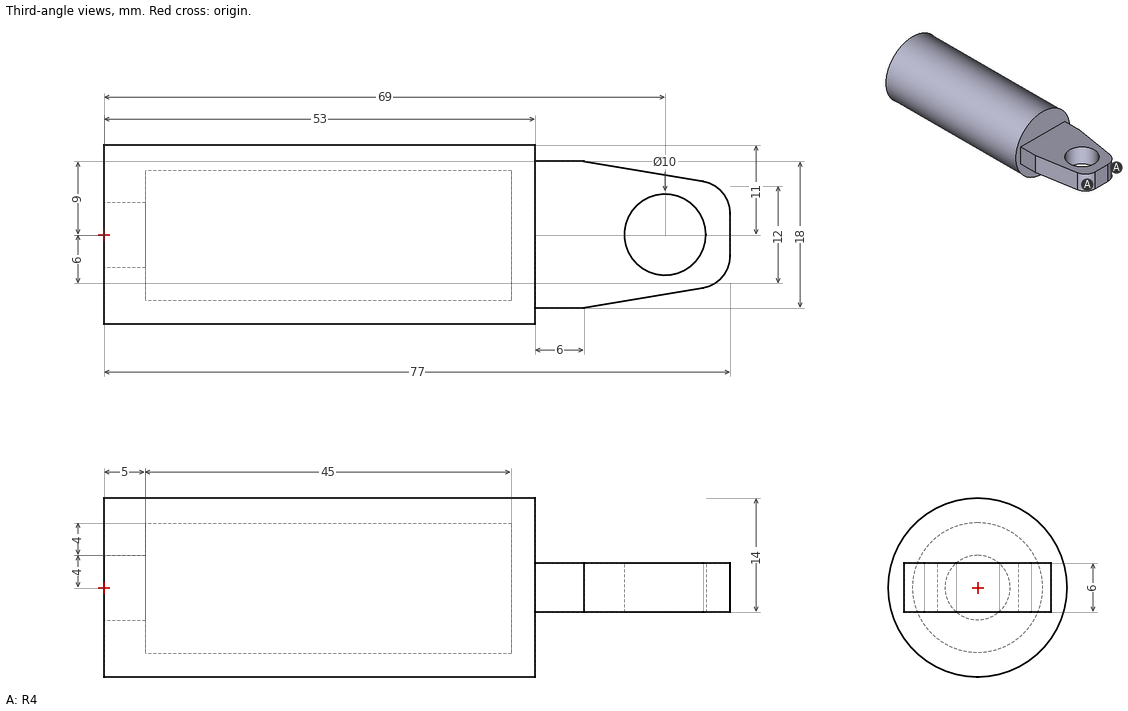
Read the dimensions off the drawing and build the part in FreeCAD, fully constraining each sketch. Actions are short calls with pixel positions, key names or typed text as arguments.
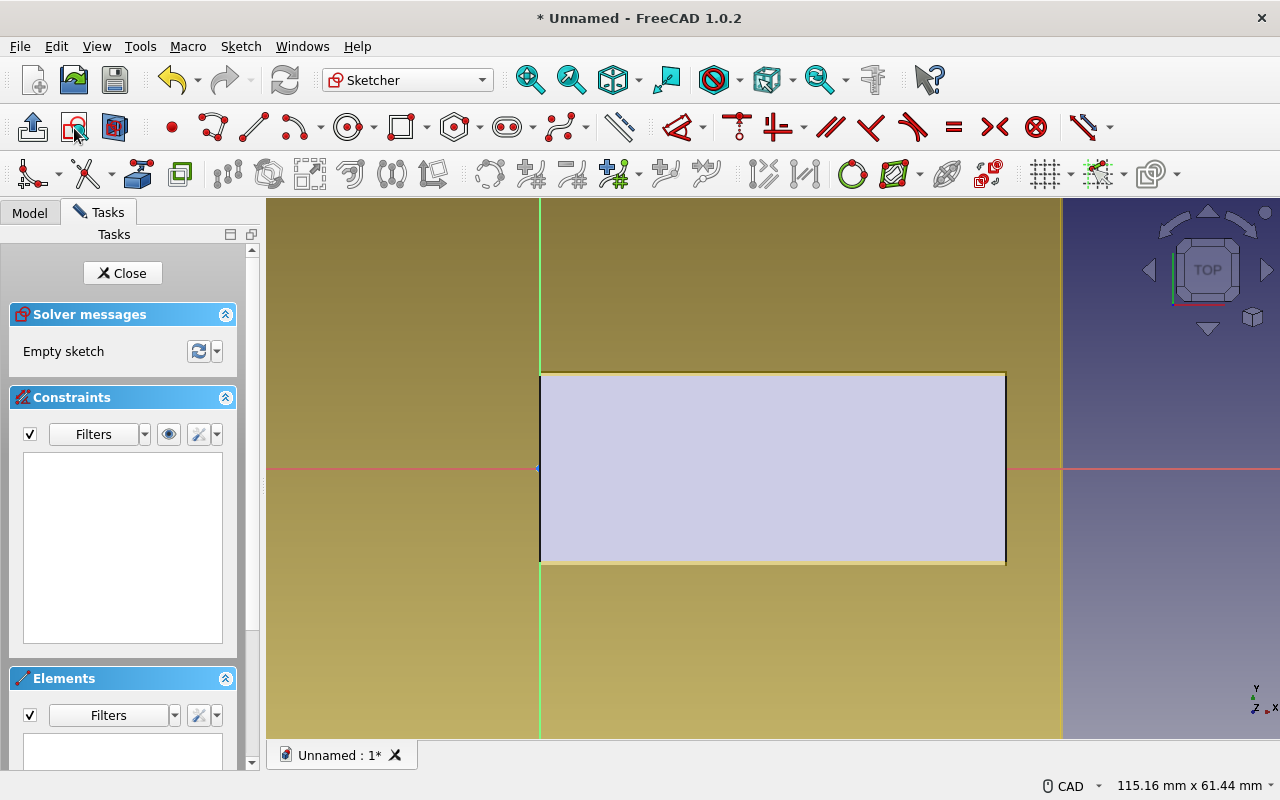
key(q)
key(s)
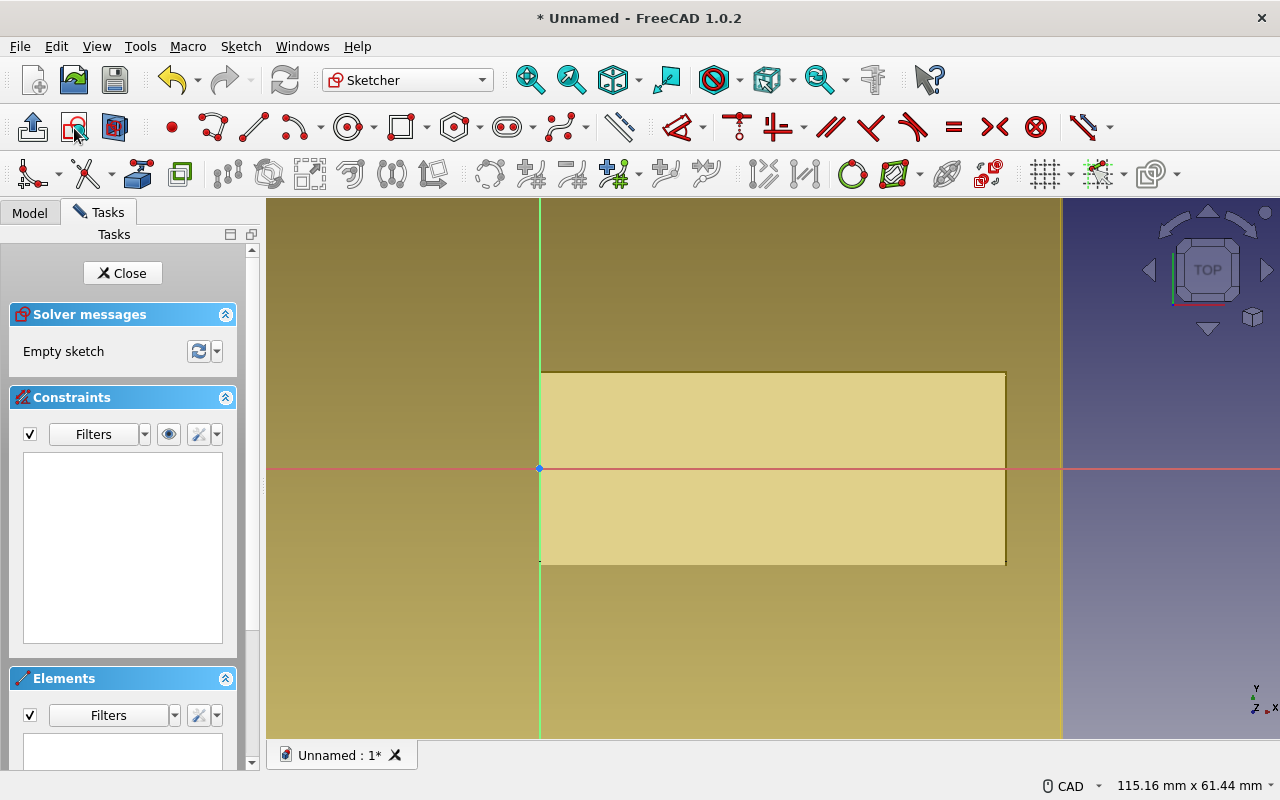
scroll(704, 468, down, 5)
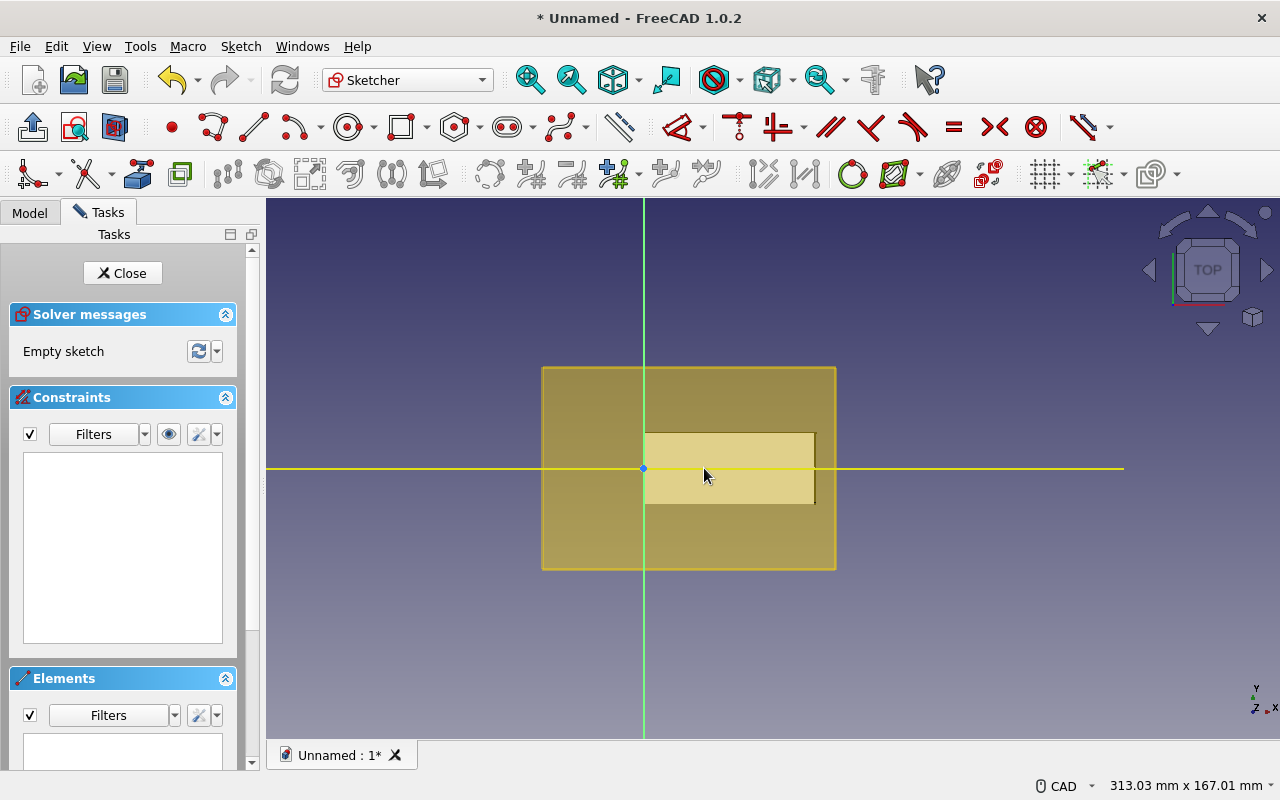
scroll(884, 469, up, 9)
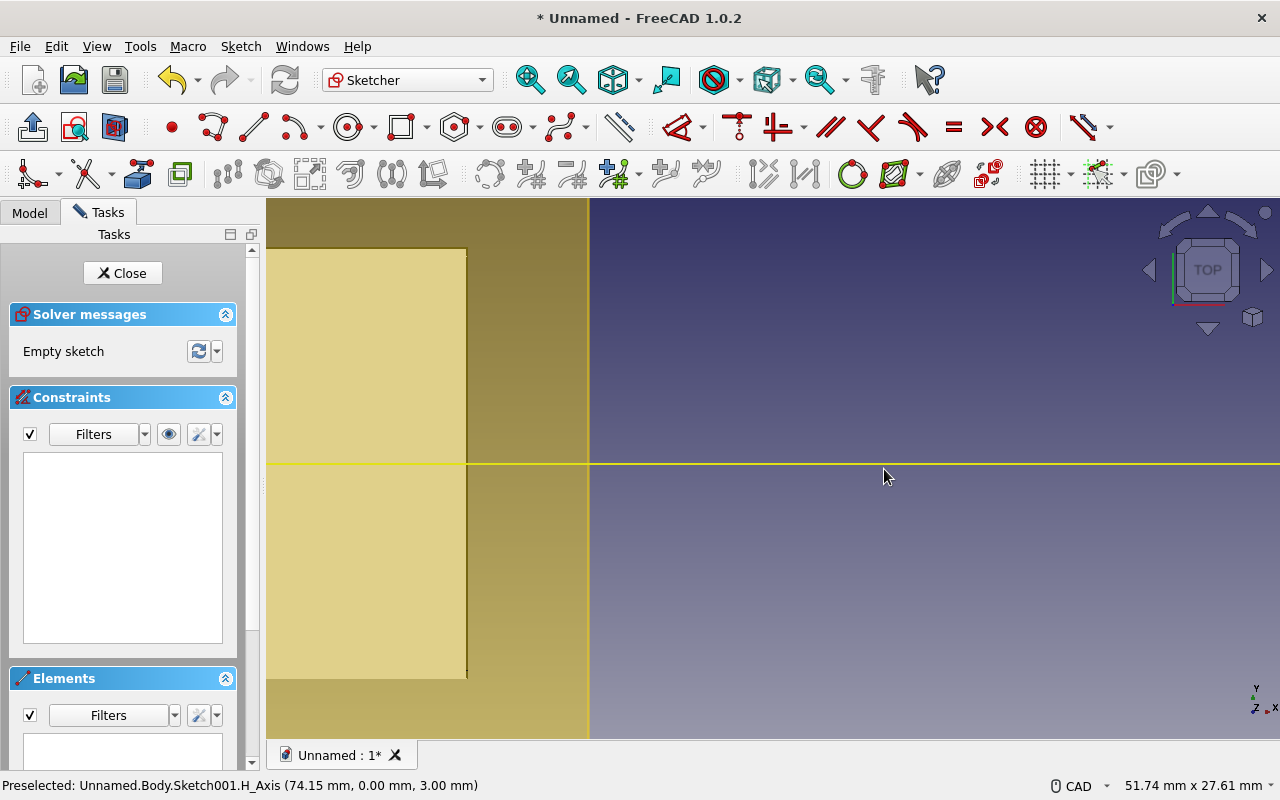
key(g)
key(m)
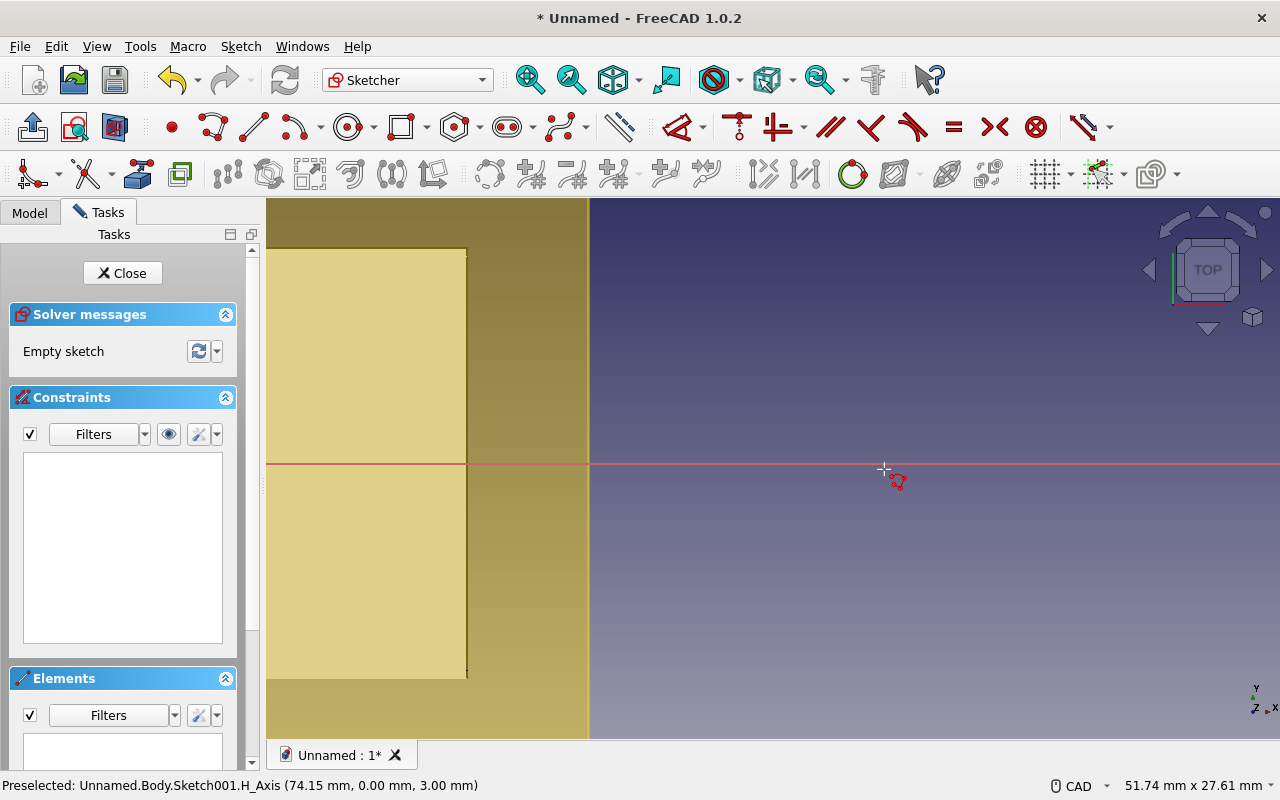
click(467, 287)
click(467, 640)
click(584, 640)
click(937, 581)
click(937, 346)
click(584, 287)
click(467, 288)
key(Escape)
key(Escape)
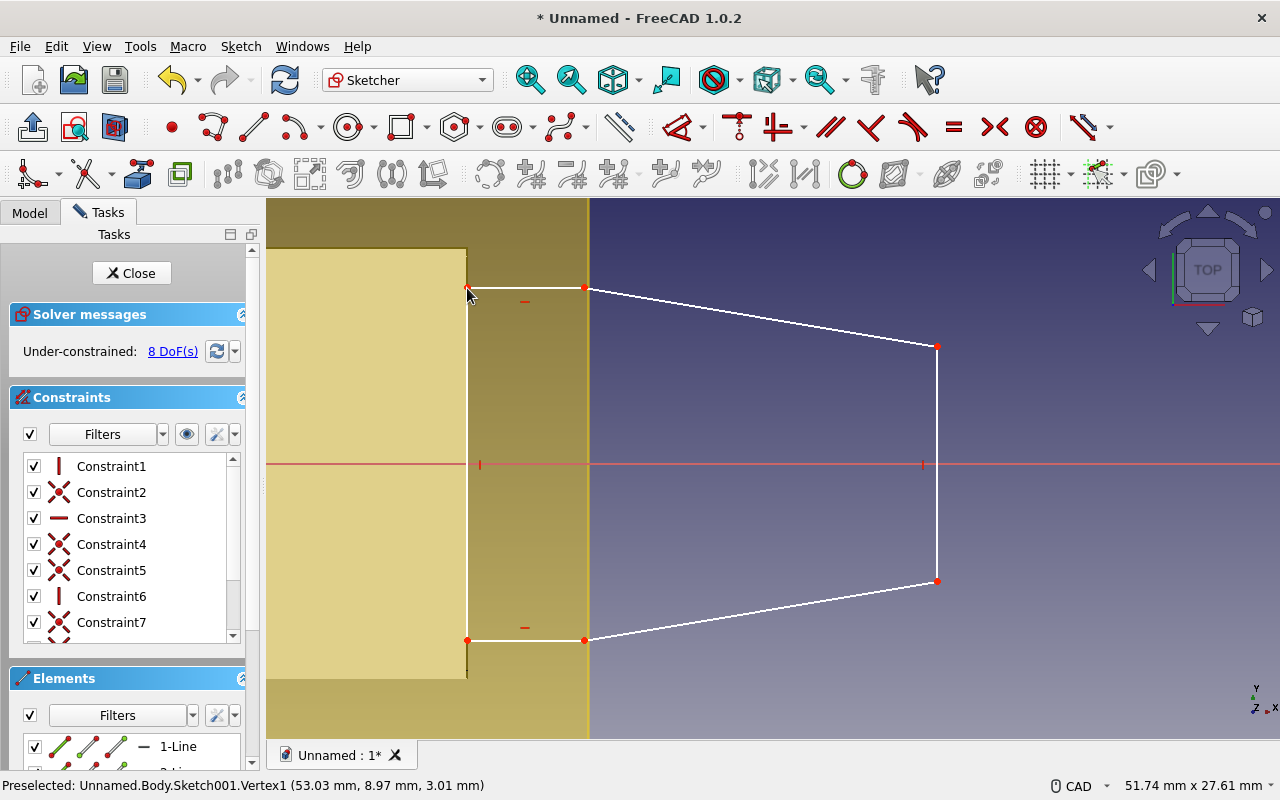
click(502, 641)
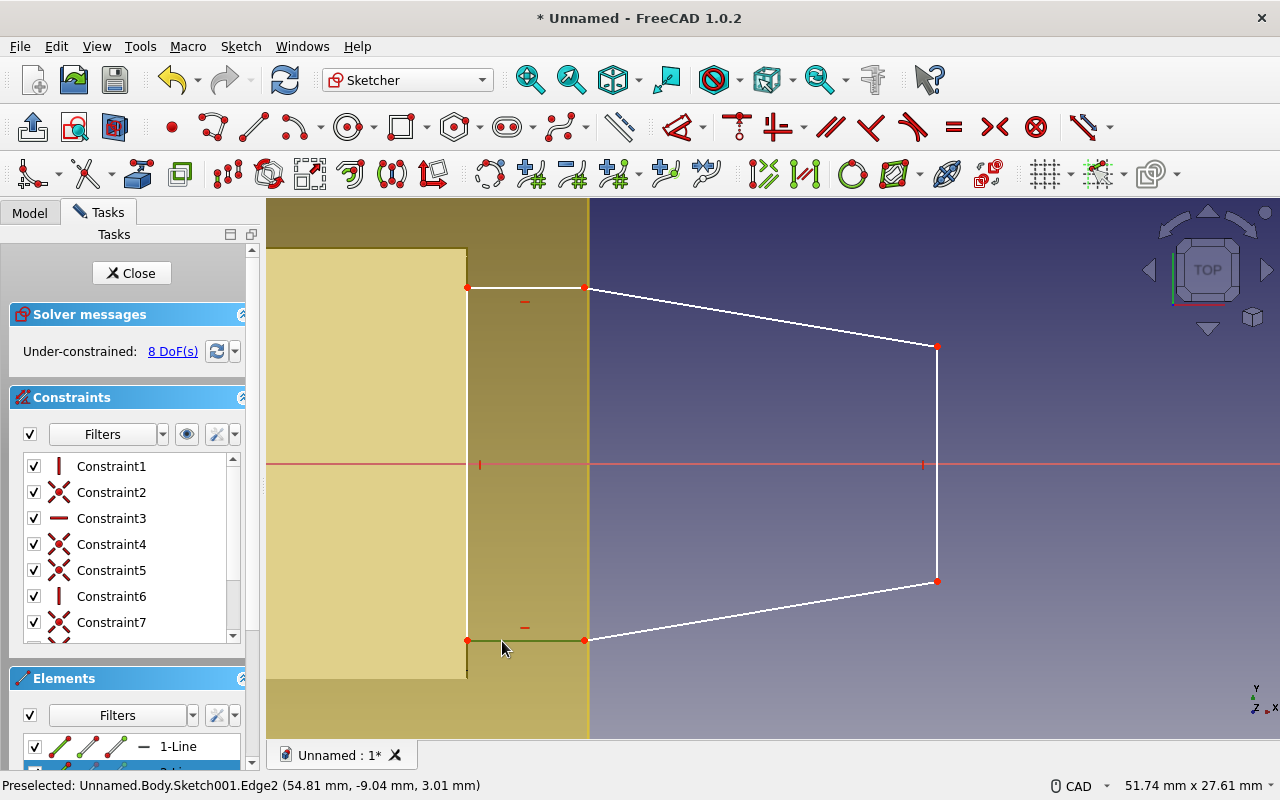
key(l)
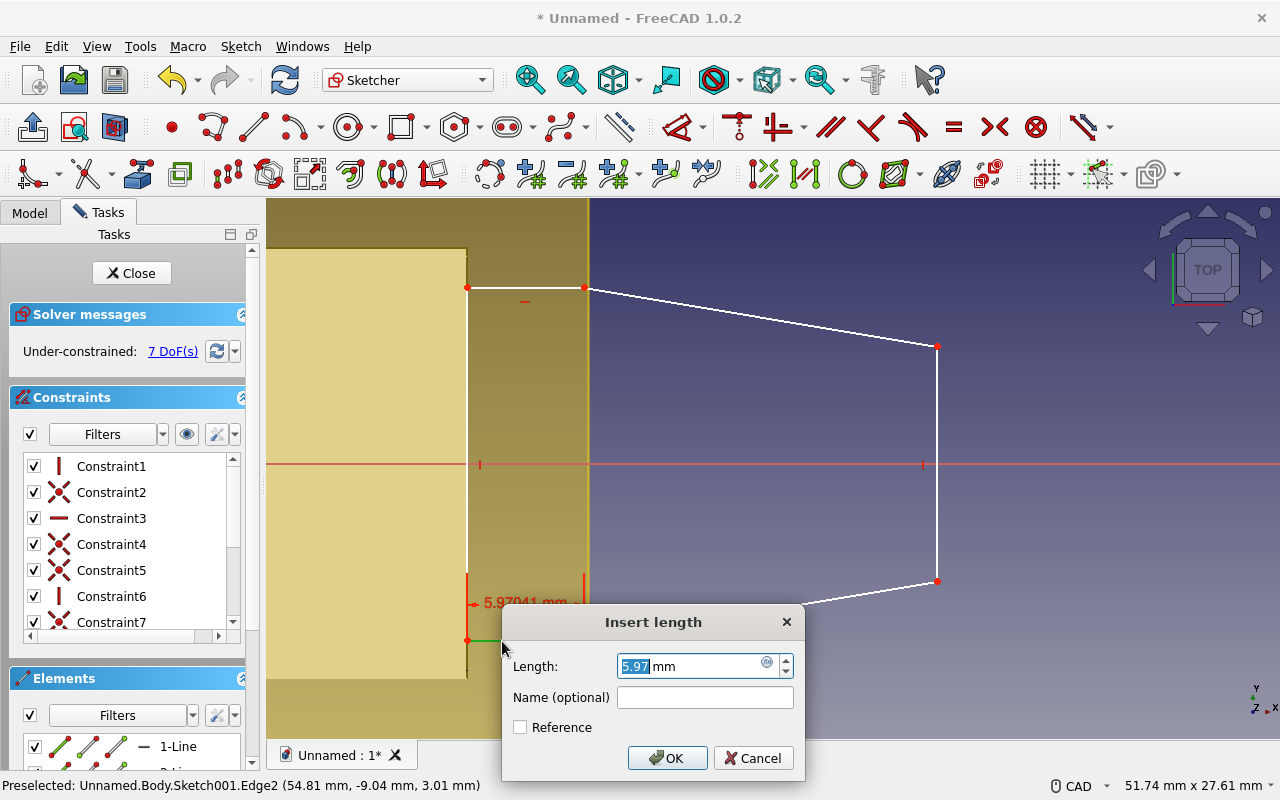
text(6)
key(Return)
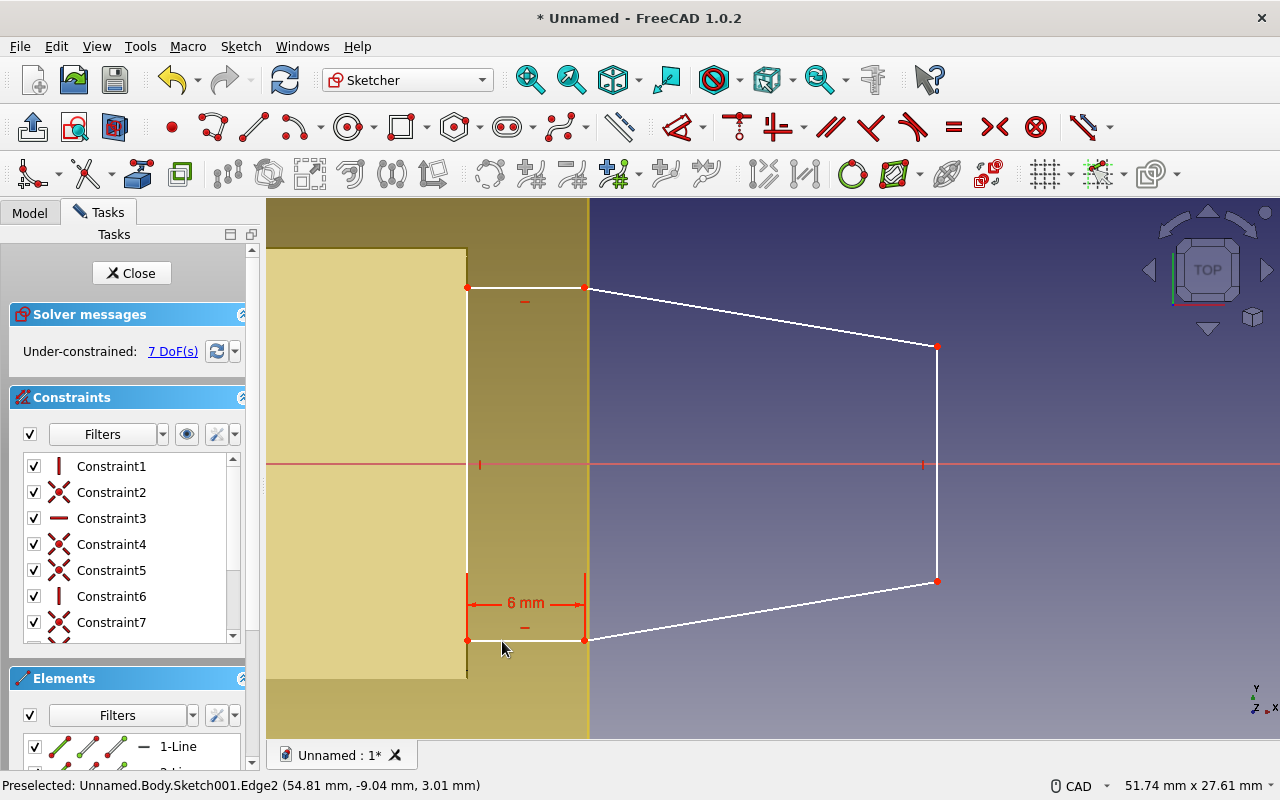
click(549, 288)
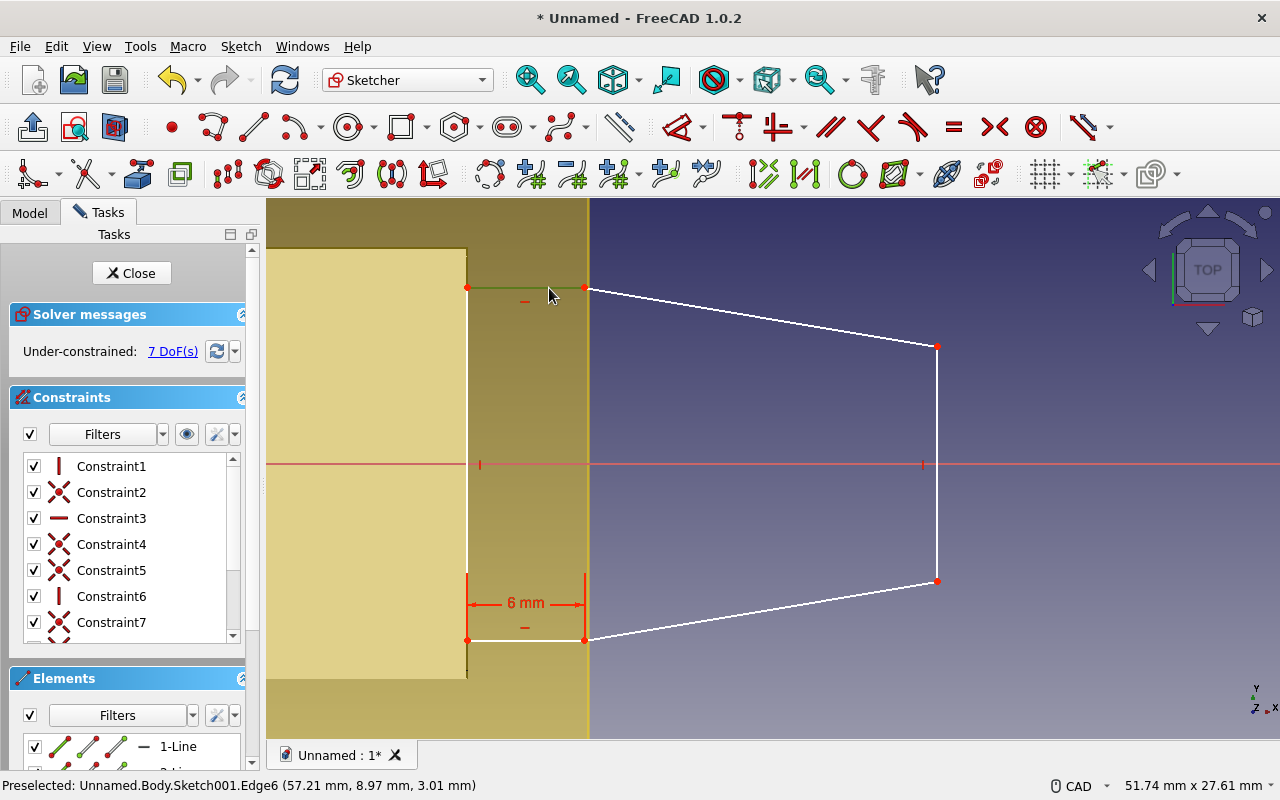
key(l)